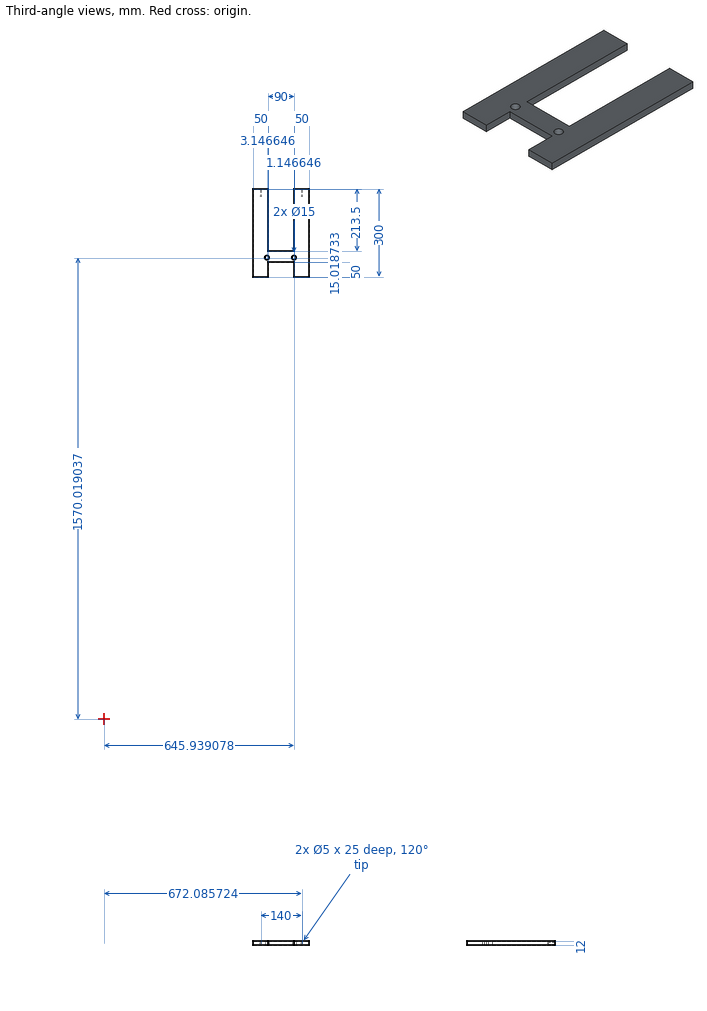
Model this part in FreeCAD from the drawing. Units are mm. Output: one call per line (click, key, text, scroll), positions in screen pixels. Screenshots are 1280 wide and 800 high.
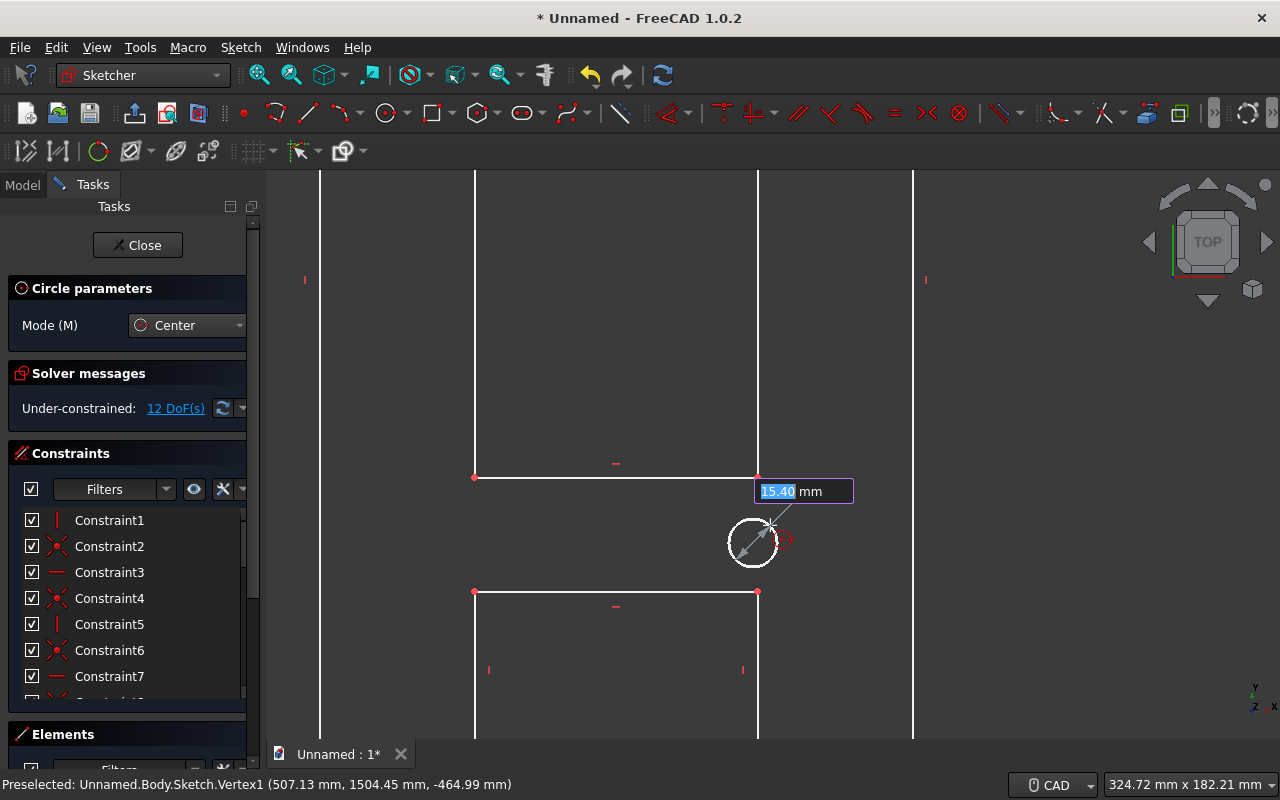
text(15)
key(Return)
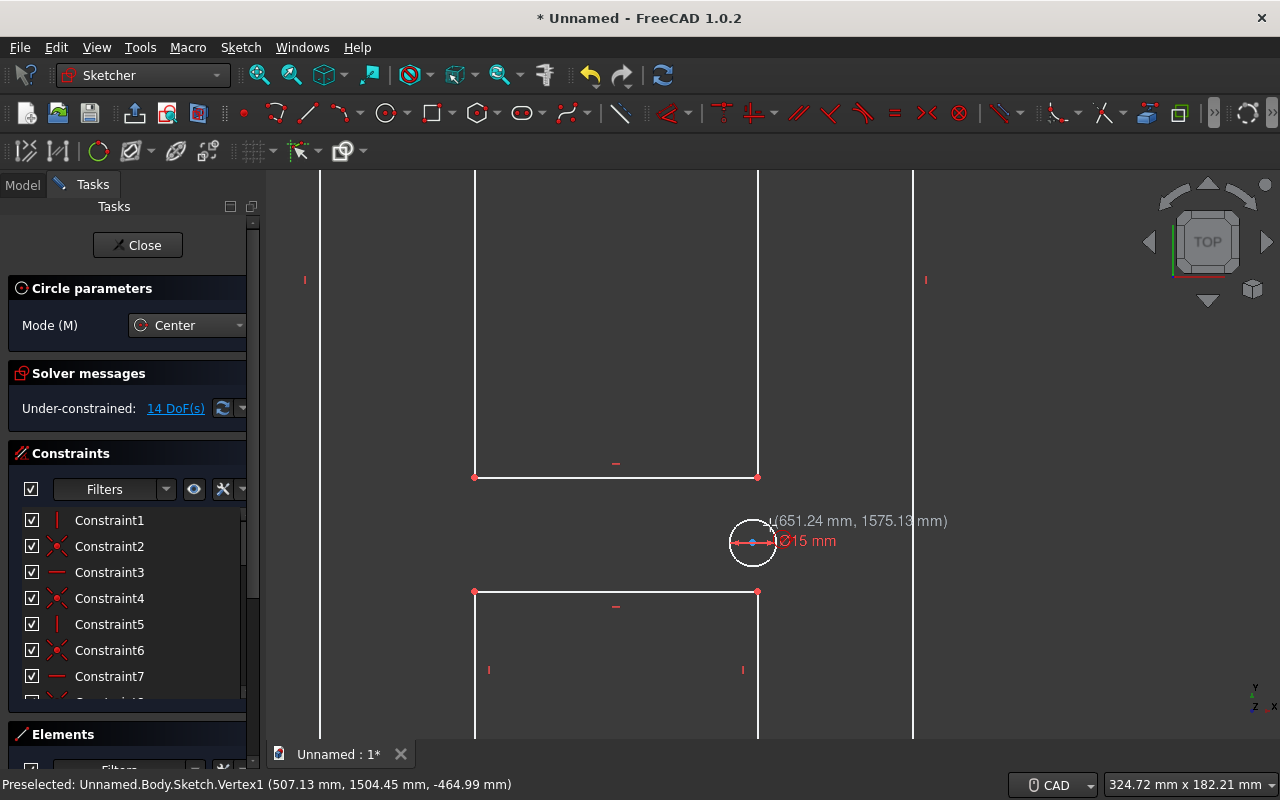
click(466, 542)
move(483, 525)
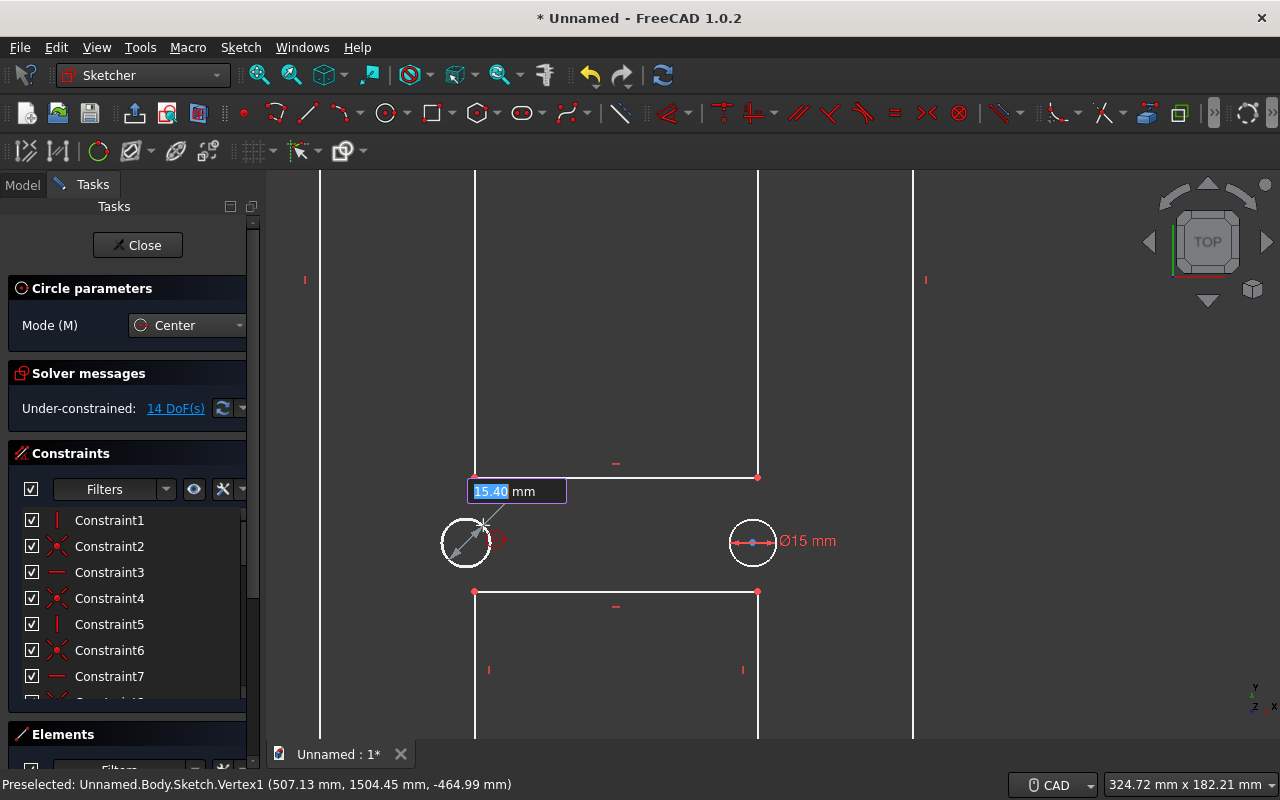
text(15)
key(Return)
key(Escape)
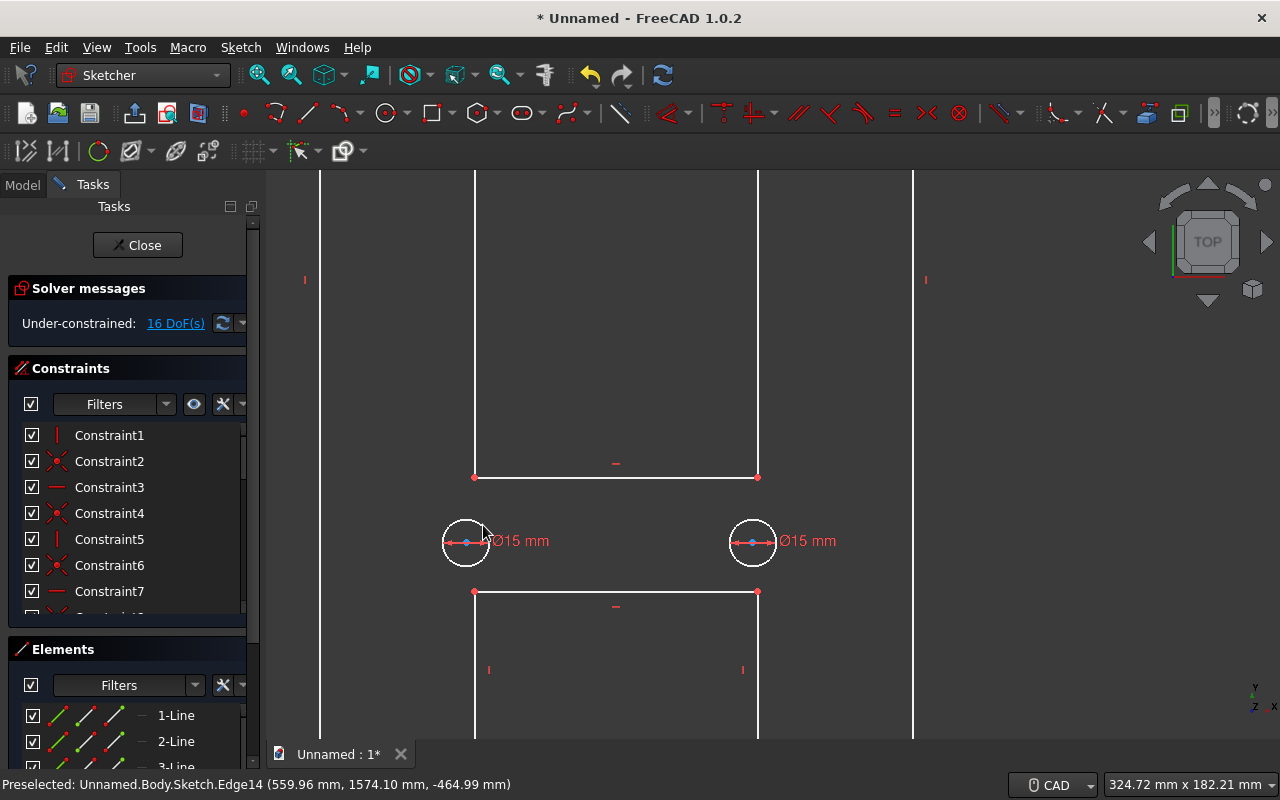
key(d)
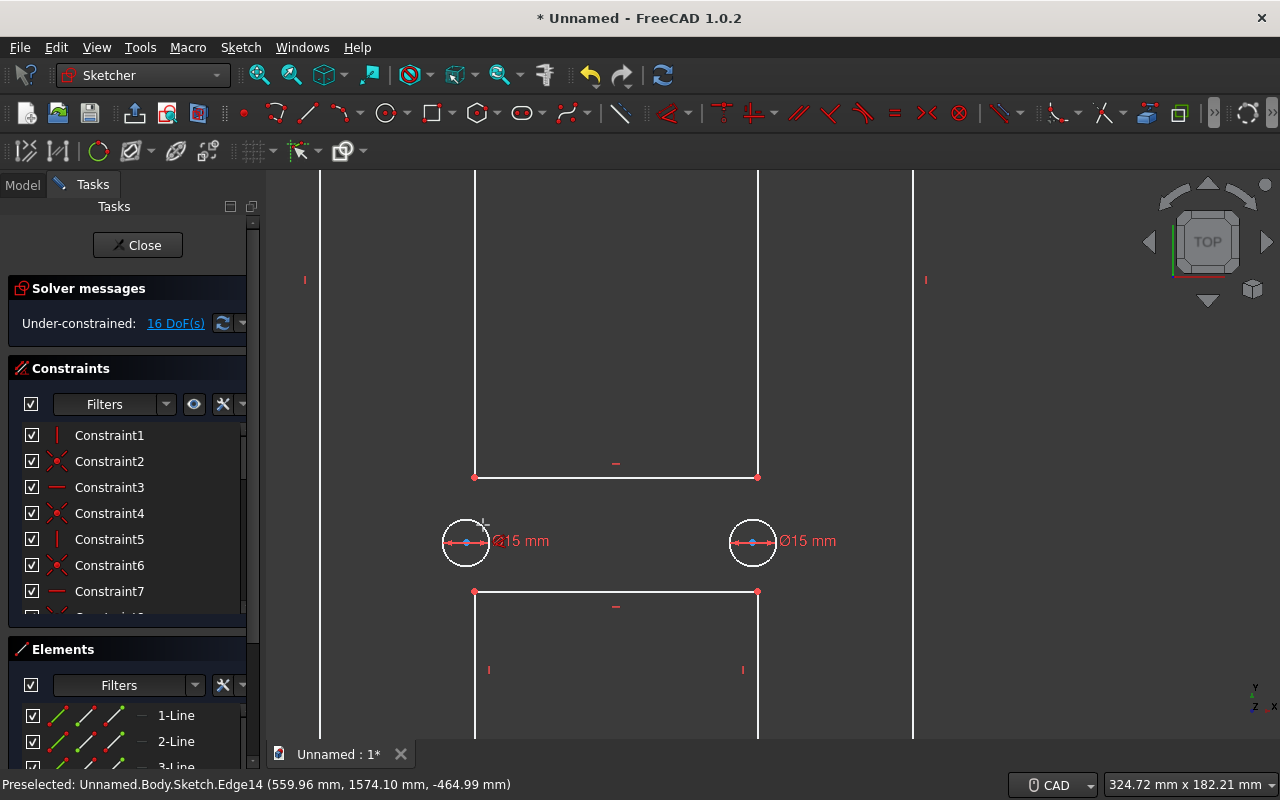
scroll(756, 558, down, 5)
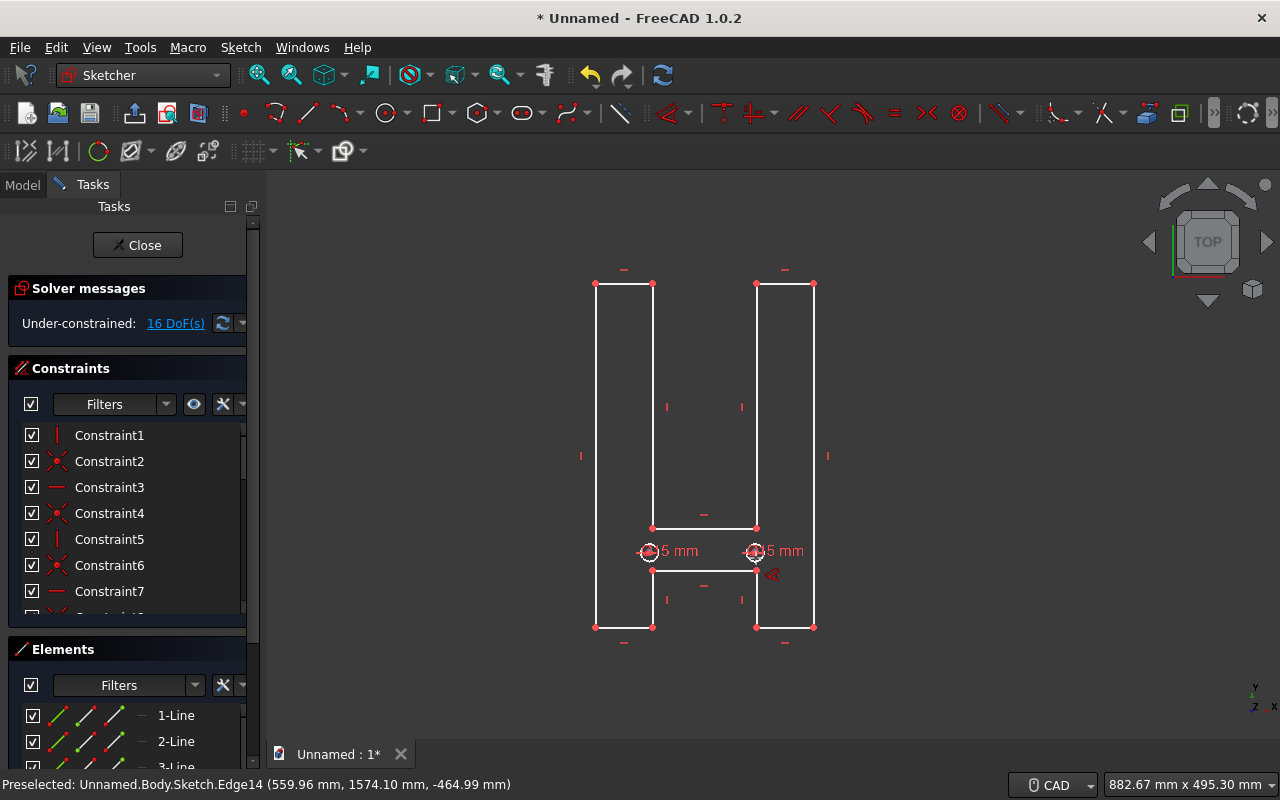
click(613, 284)
click(624, 250)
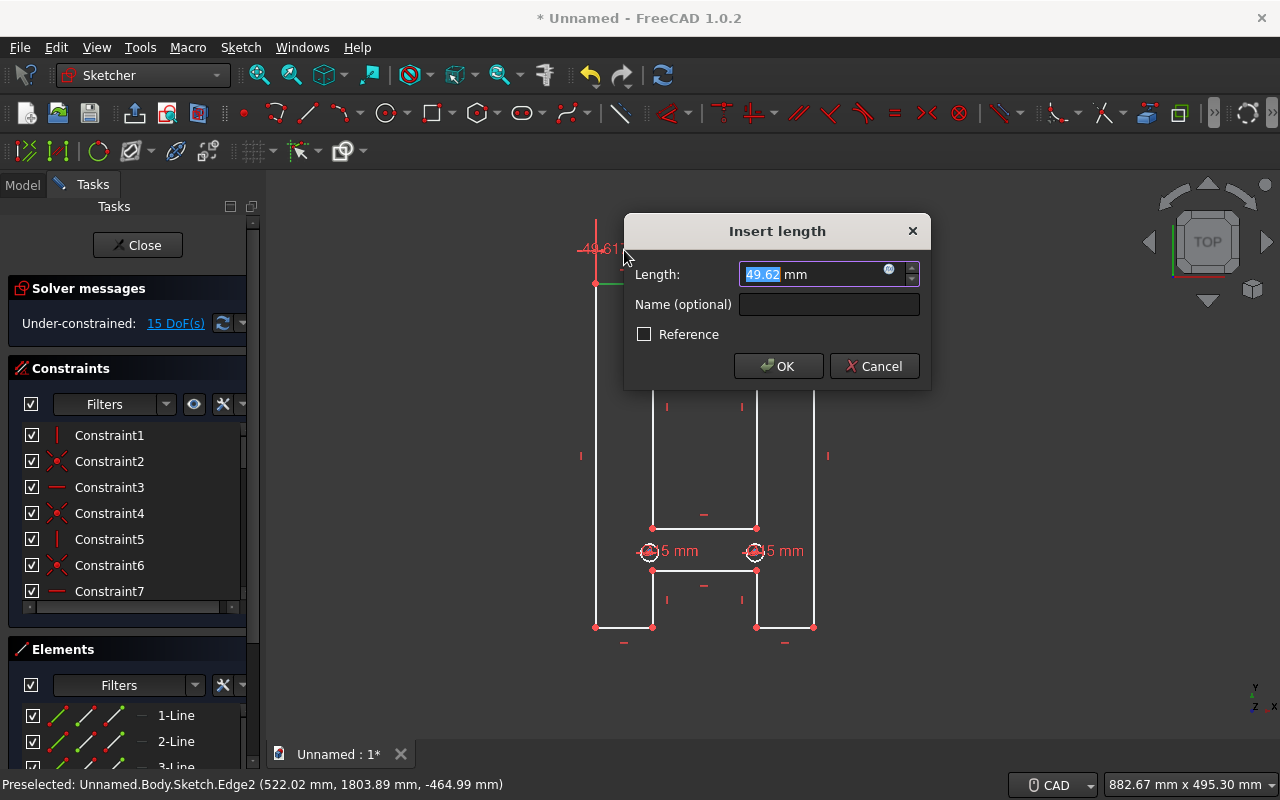
text(50)
key(Return)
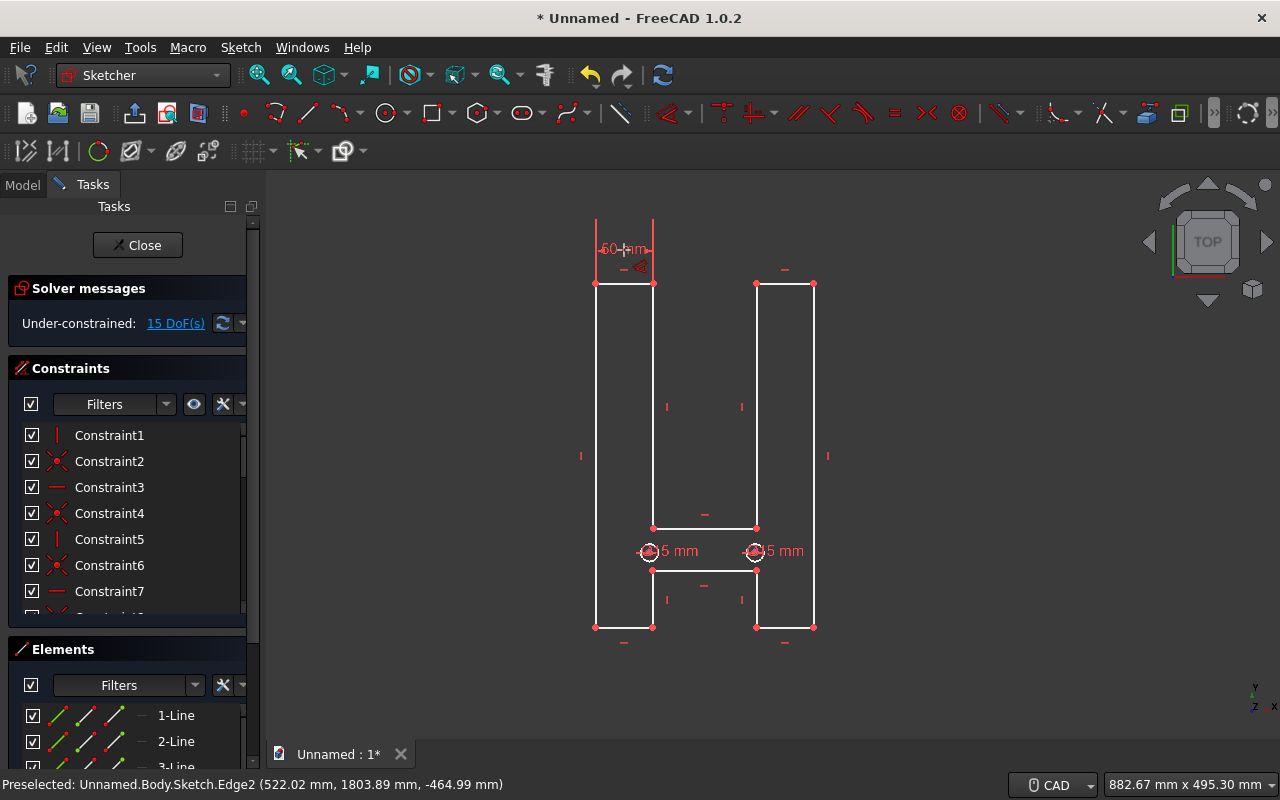
click(684, 529)
click(705, 495)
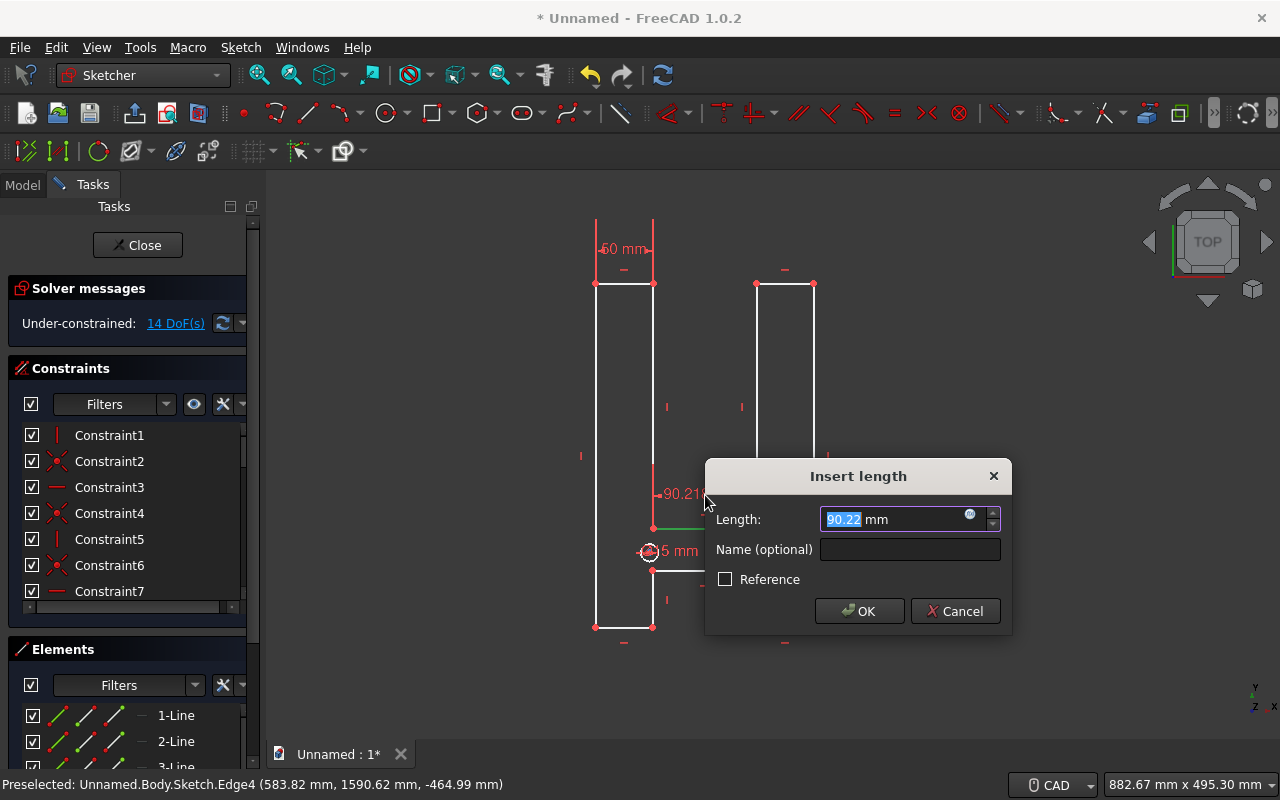
text(90)
key(Return)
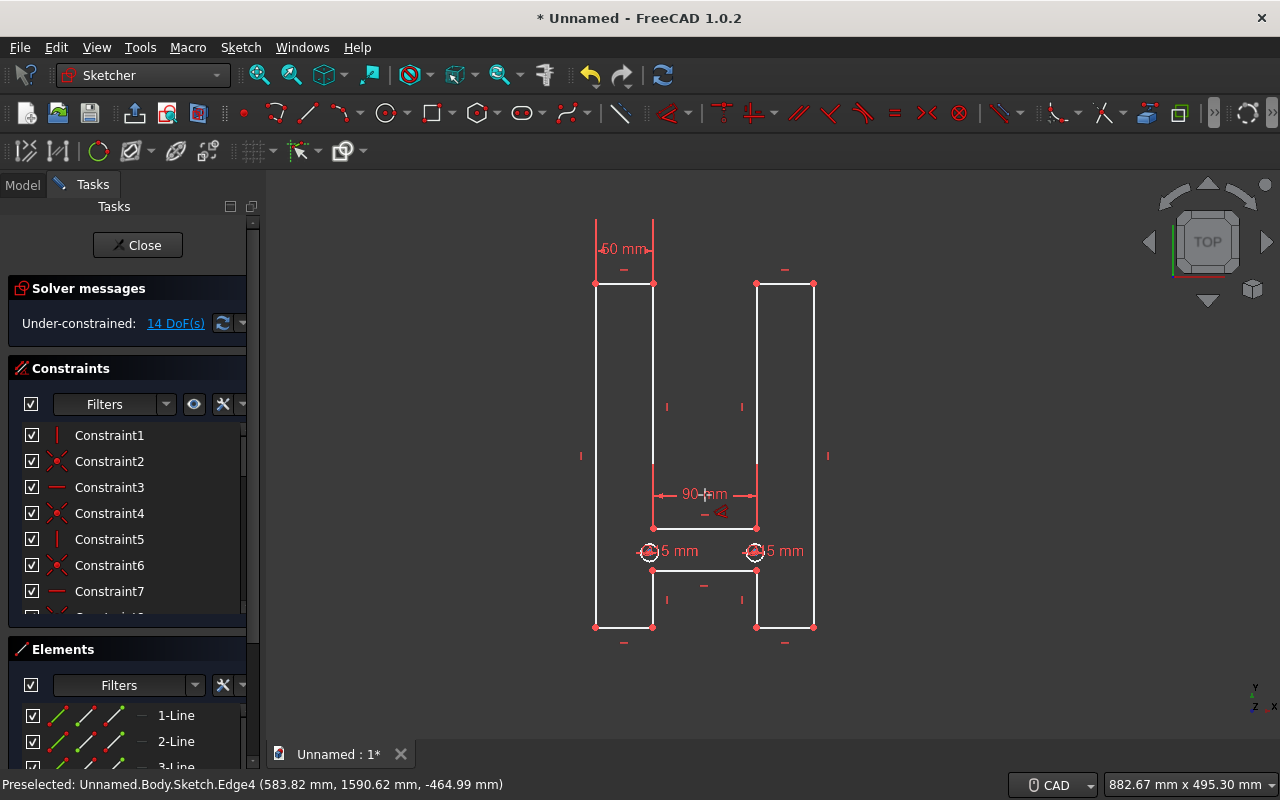
click(774, 284)
click(785, 250)